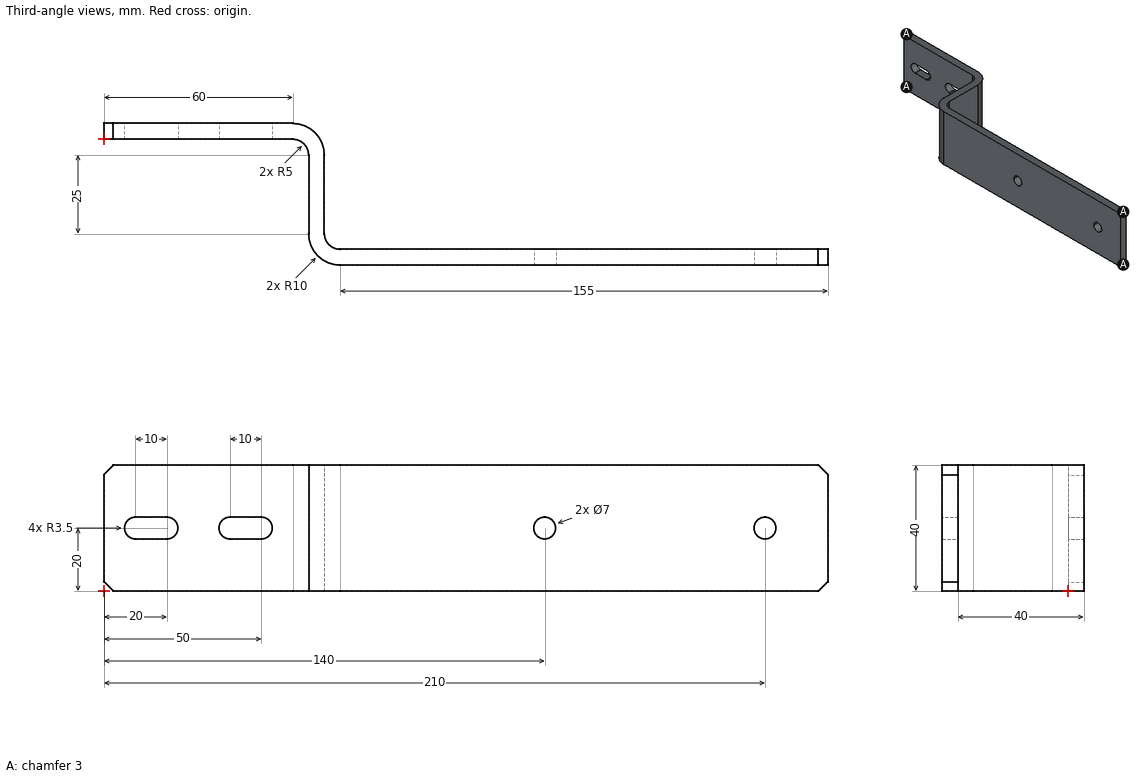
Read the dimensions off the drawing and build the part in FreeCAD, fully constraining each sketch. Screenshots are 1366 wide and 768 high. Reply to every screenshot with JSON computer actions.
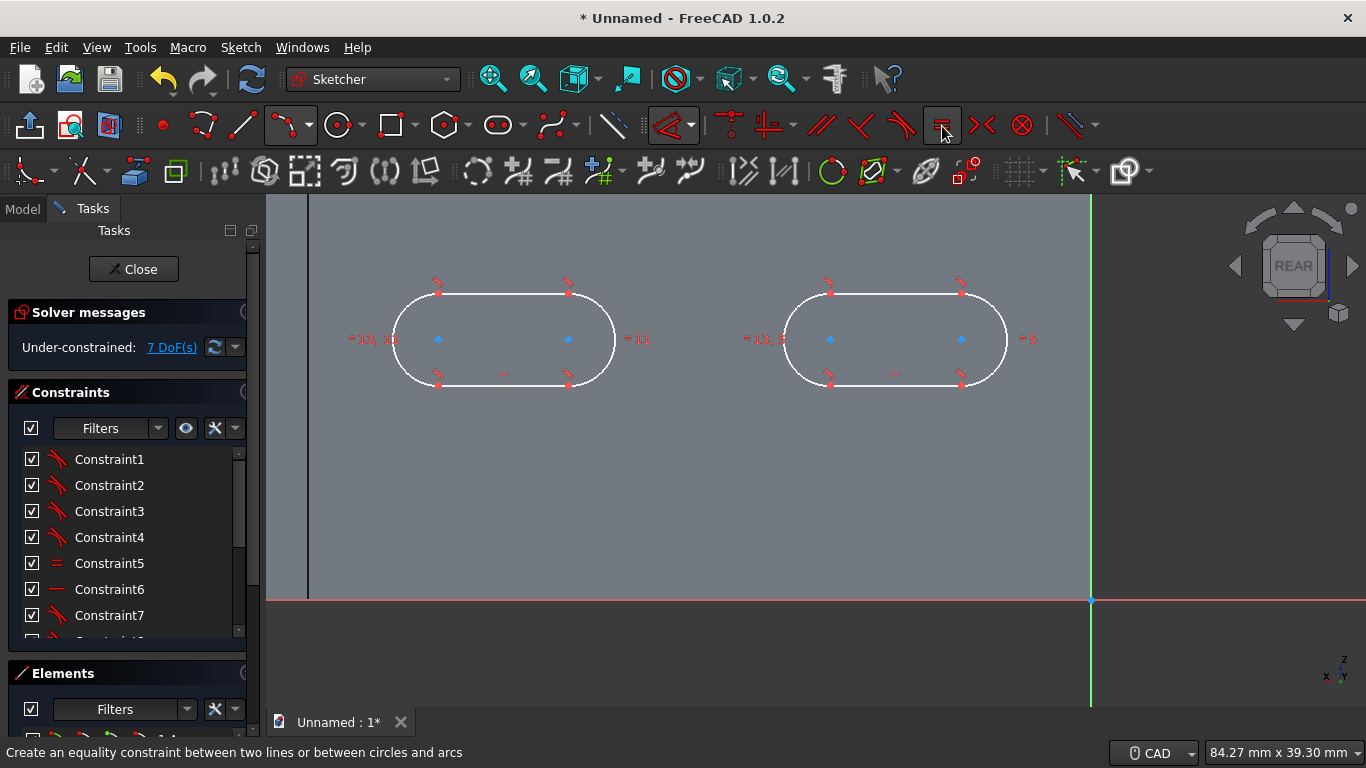
{"action": "left_click", "coordinate": [793, 313]}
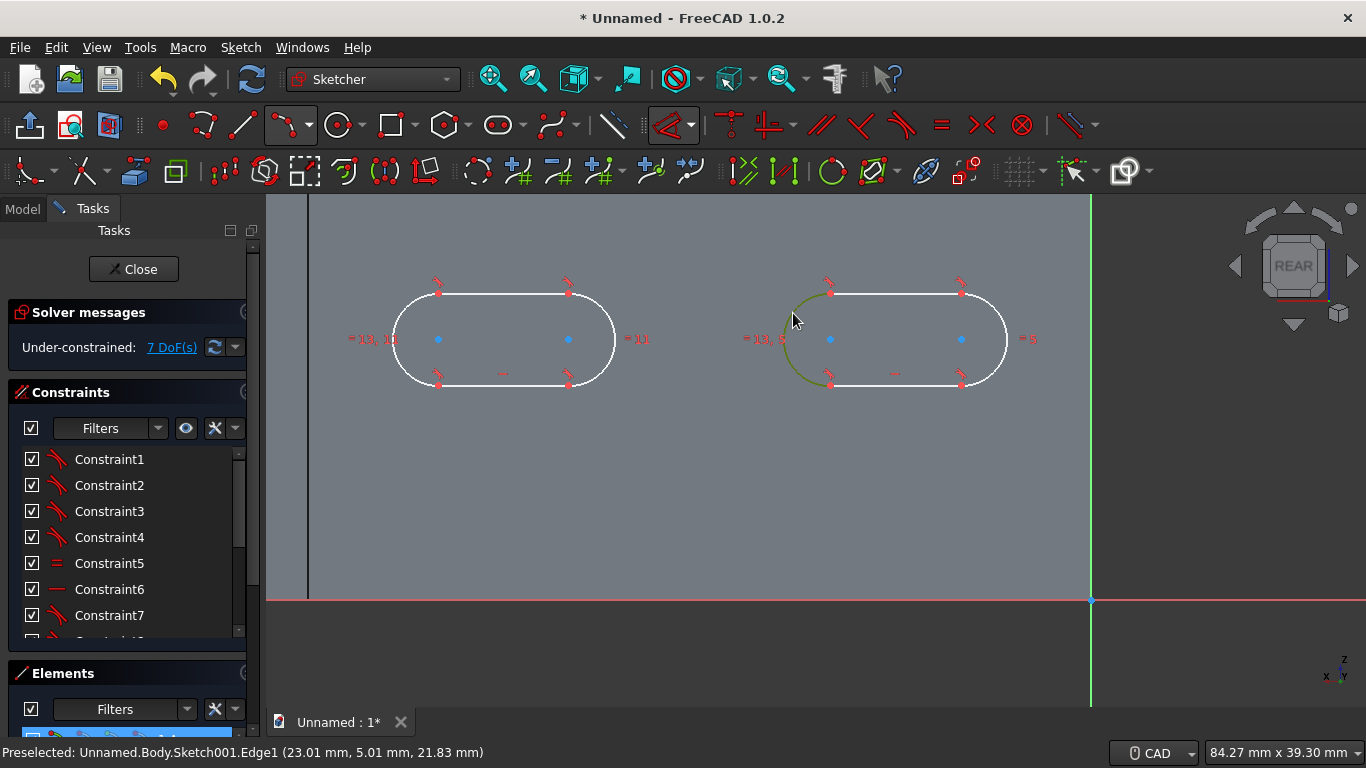
{"action": "key", "text": "k r"}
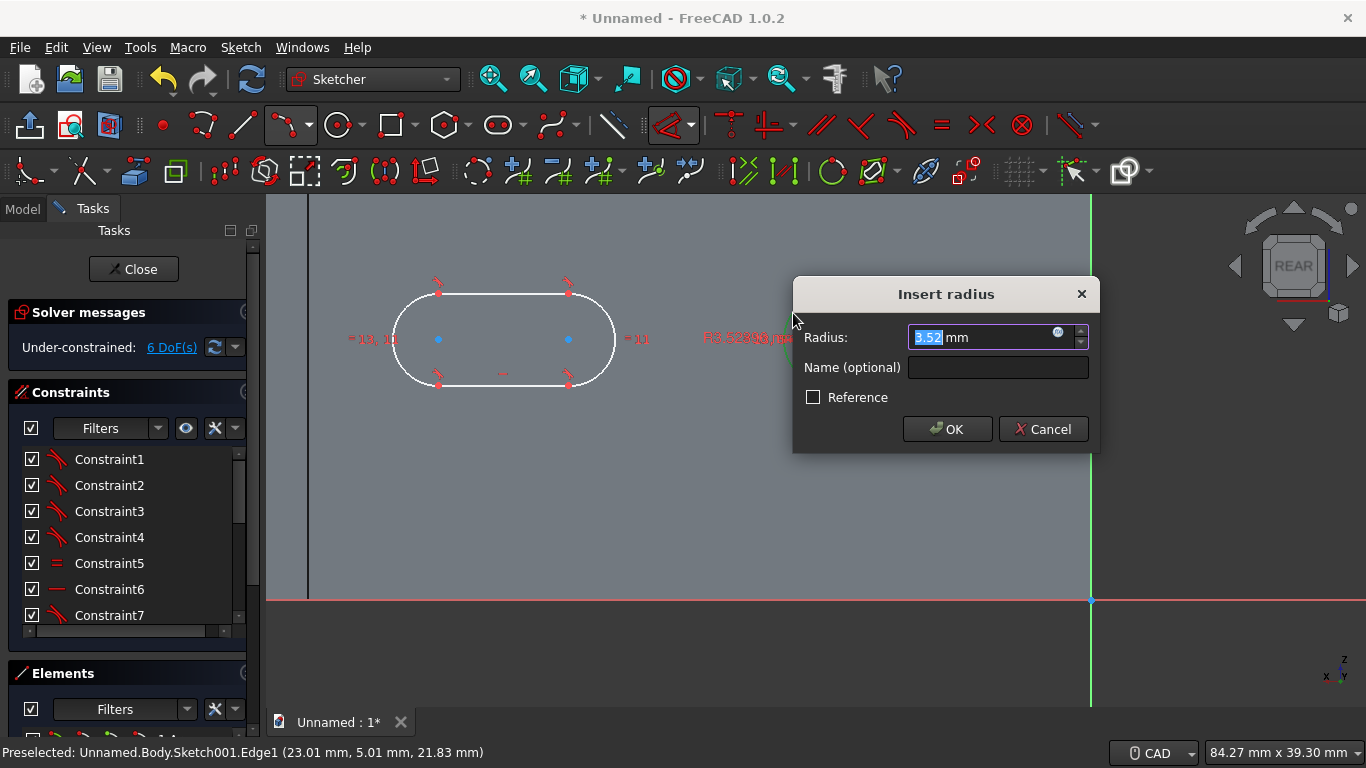
{"action": "type", "text": "3.5"}
{"action": "key", "text": "Return"}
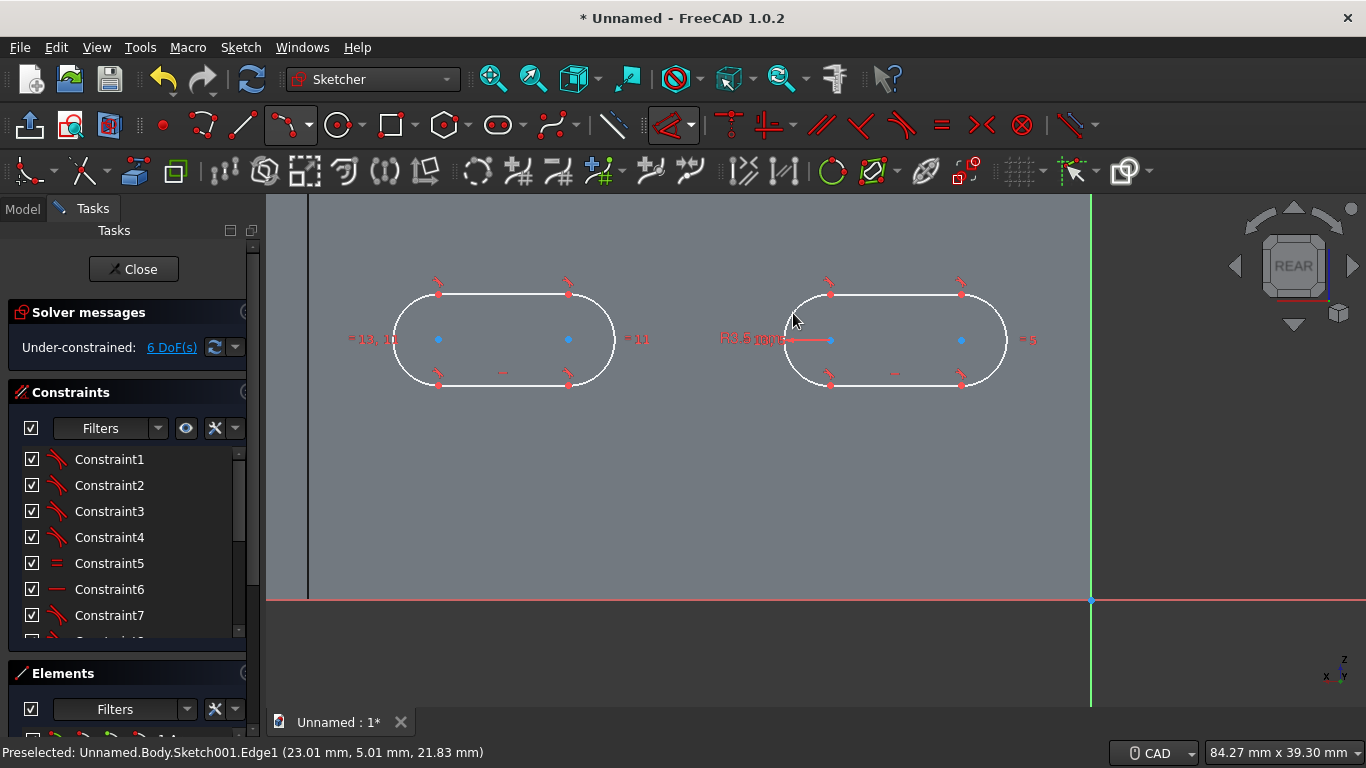
{"action": "left_click", "coordinate": [869, 295]}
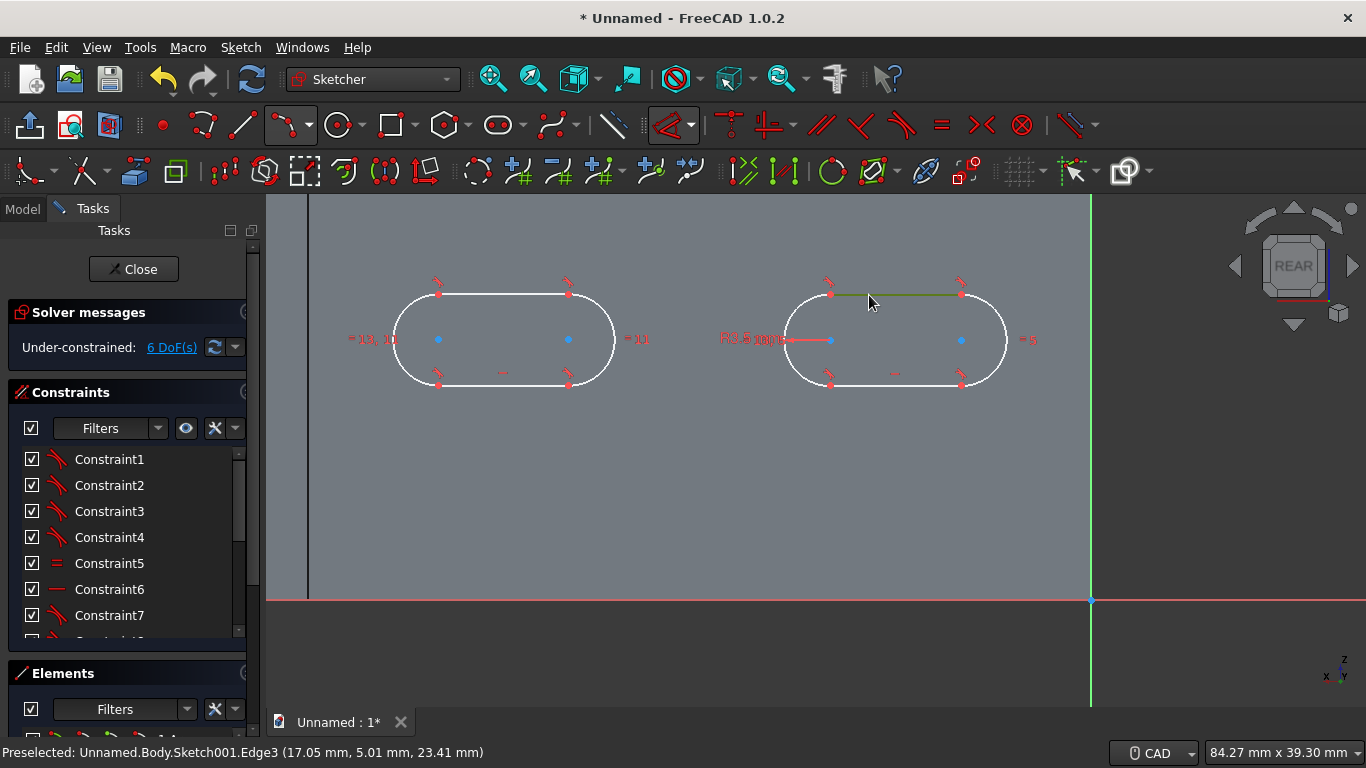
{"action": "left_click", "coordinate": [694, 126]}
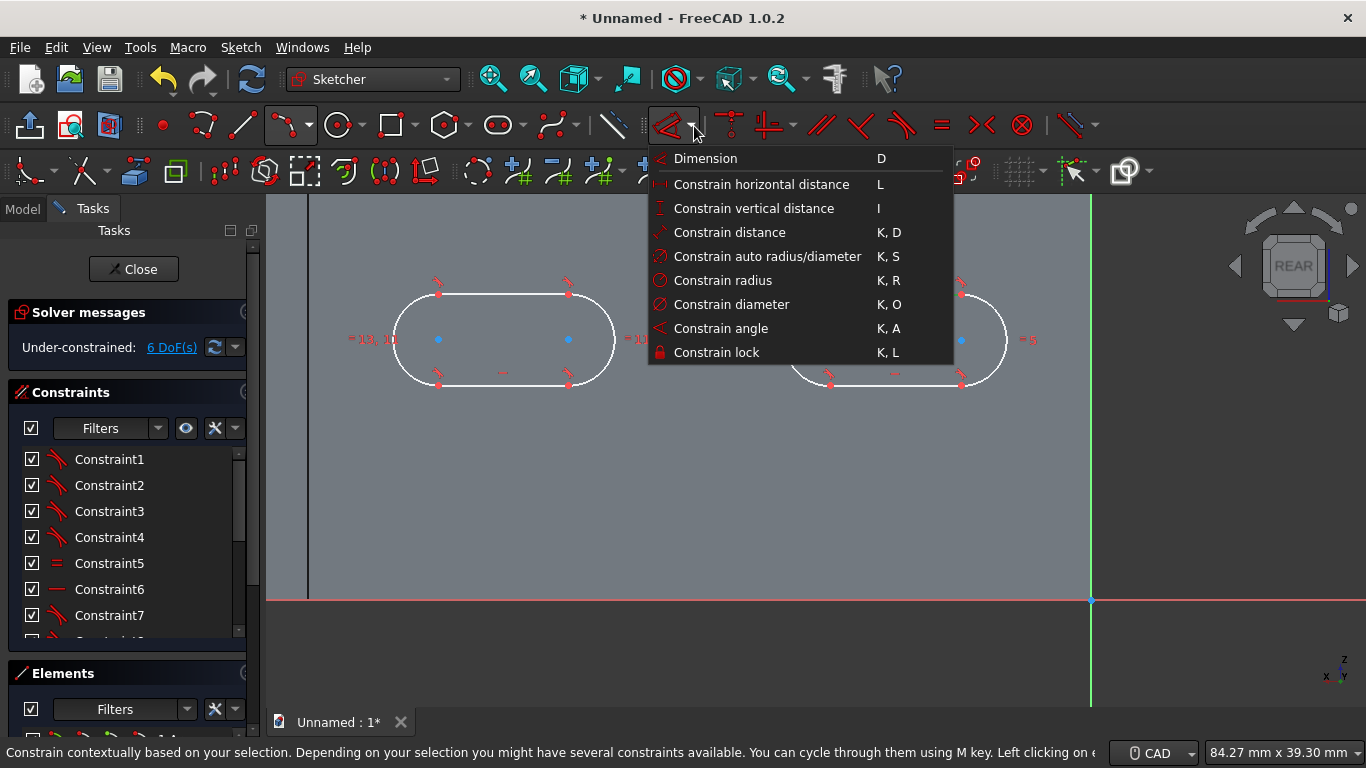
{"action": "left_click", "coordinate": [801, 184]}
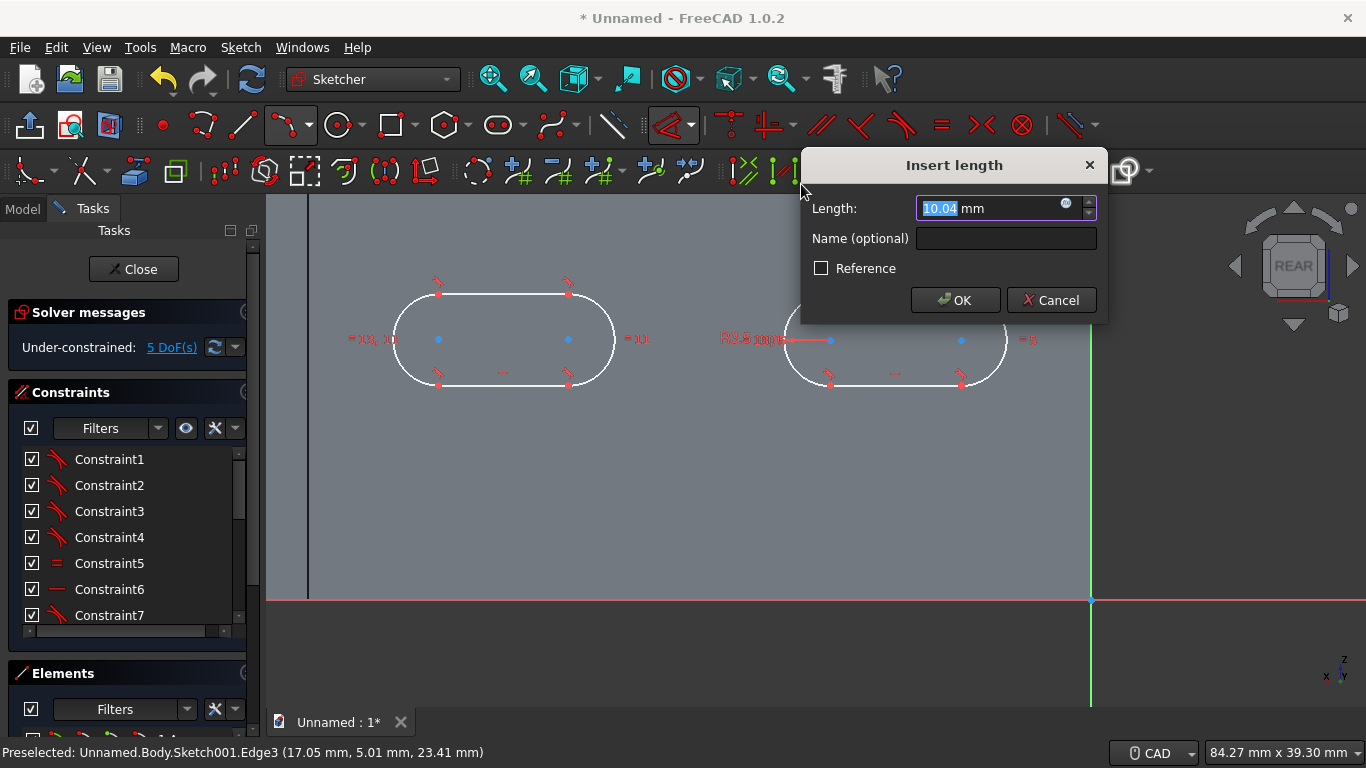
{"action": "type", "text": "10"}
{"action": "key", "text": "Return"}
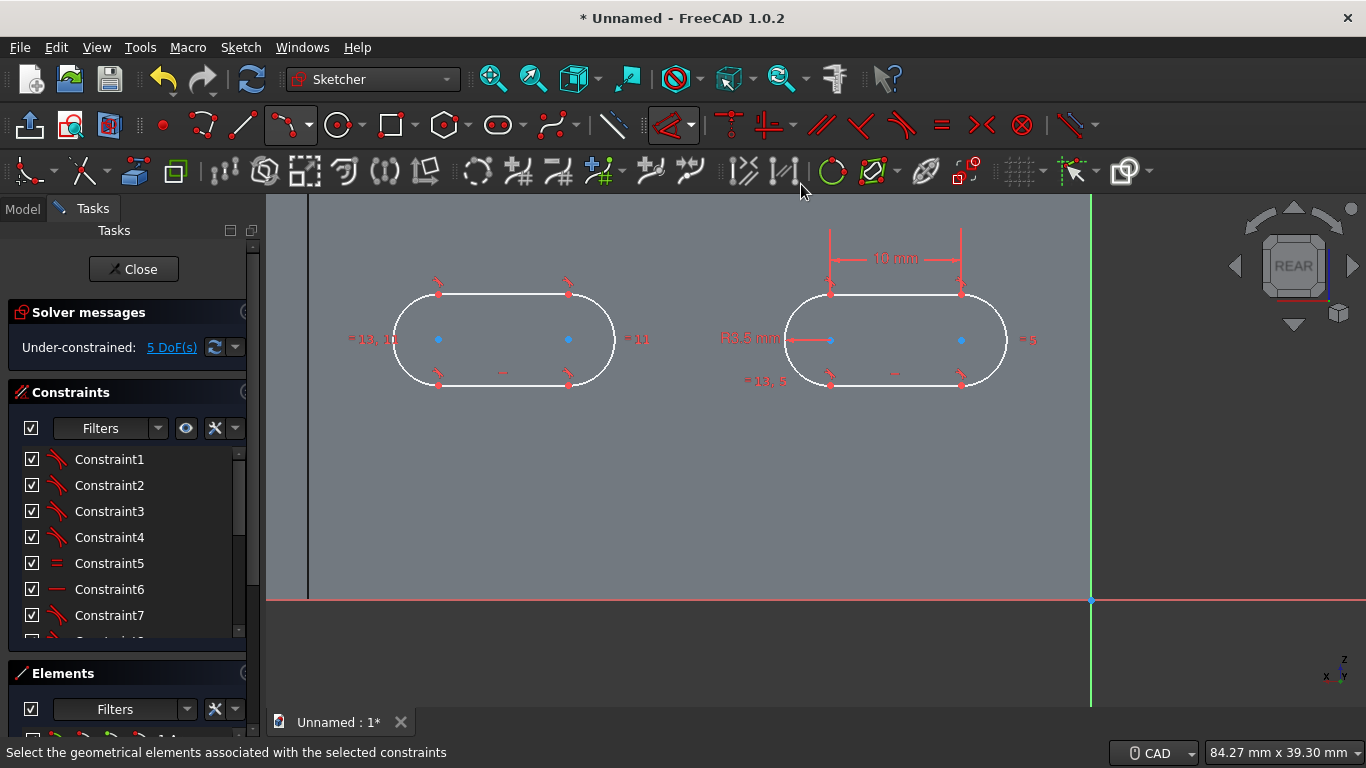
{"action": "left_click", "coordinate": [478, 294]}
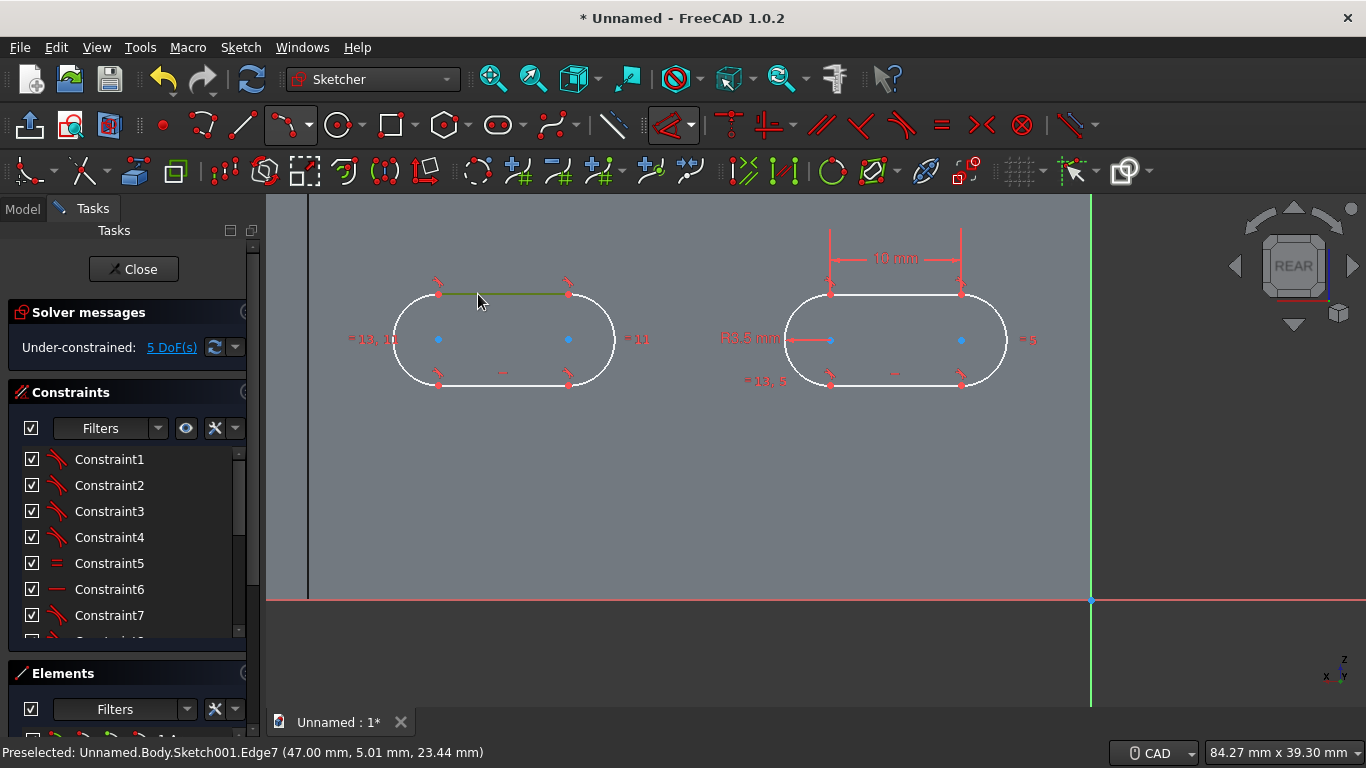
{"action": "key", "text": "l"}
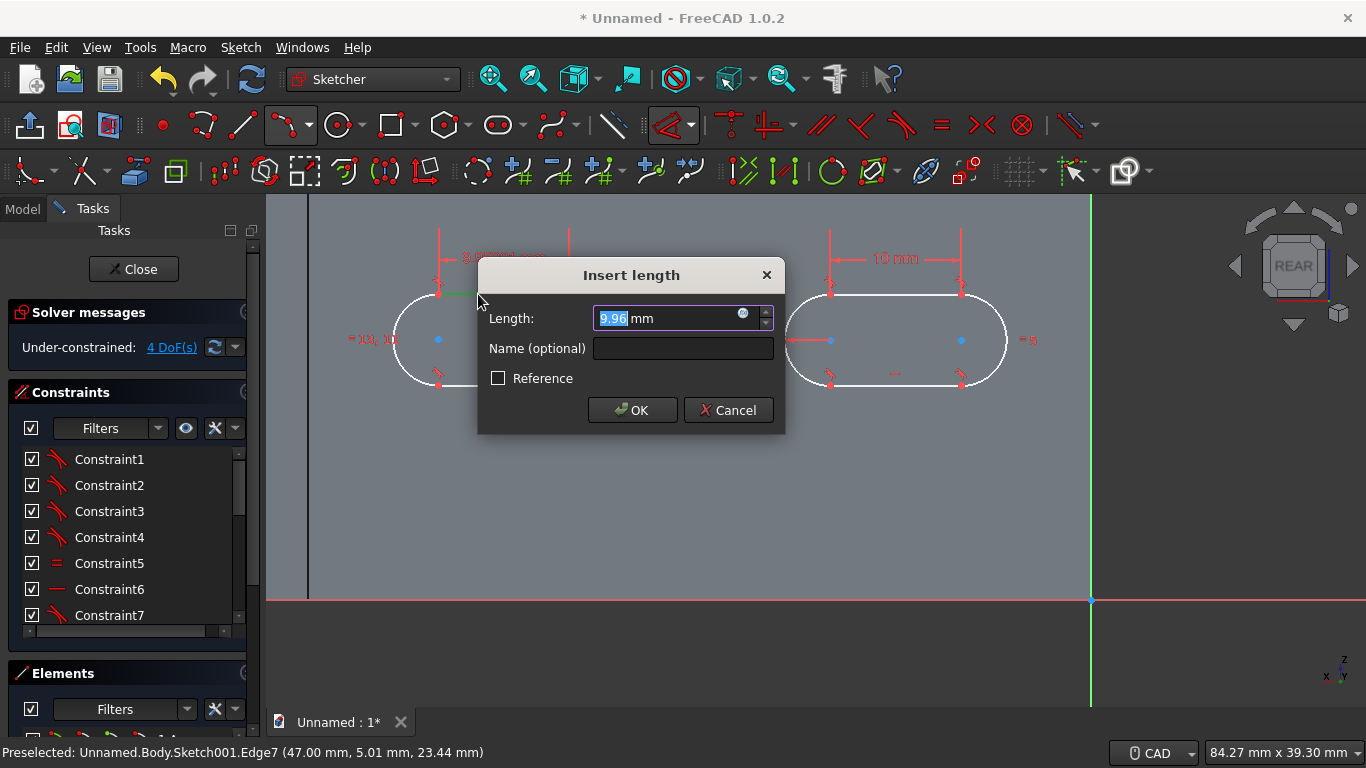
{"action": "type", "text": "10"}
{"action": "key", "text": "Return"}